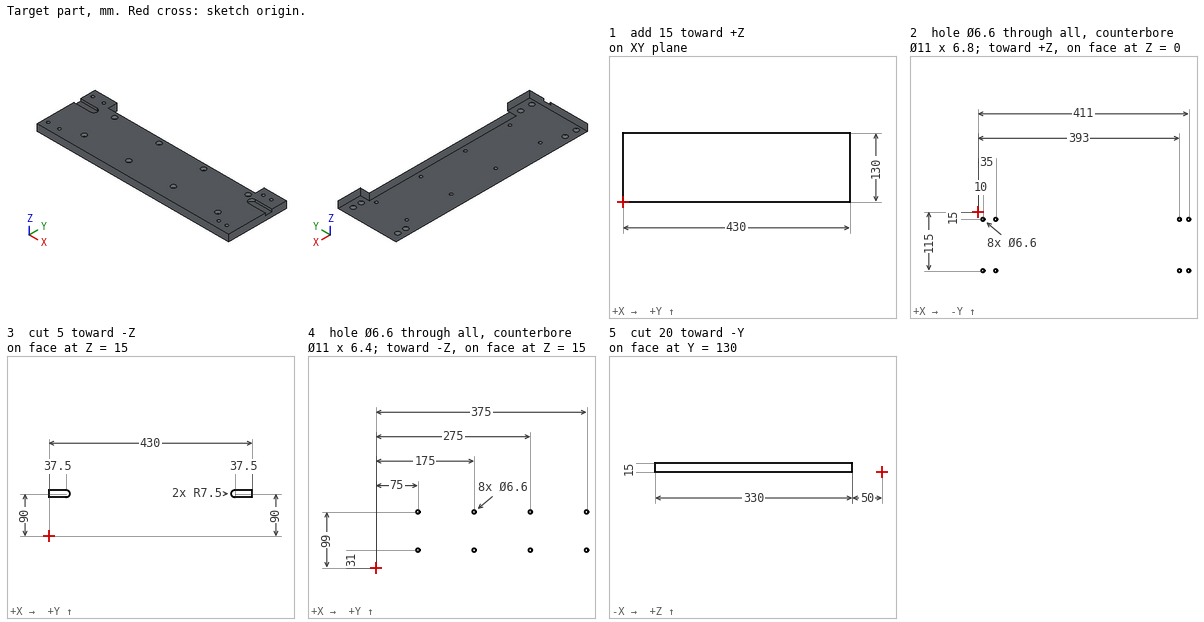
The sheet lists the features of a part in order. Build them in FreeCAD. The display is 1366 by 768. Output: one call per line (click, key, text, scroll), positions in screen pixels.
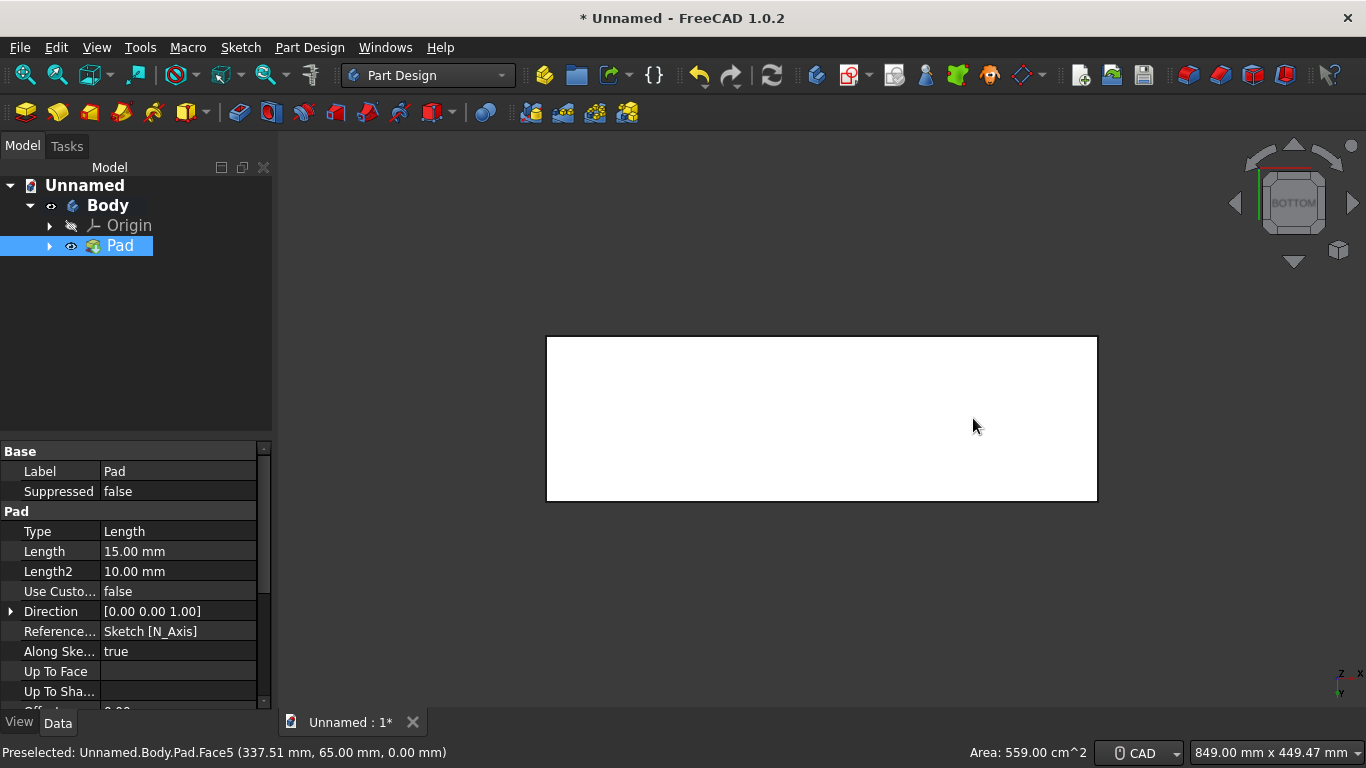
click(850, 76)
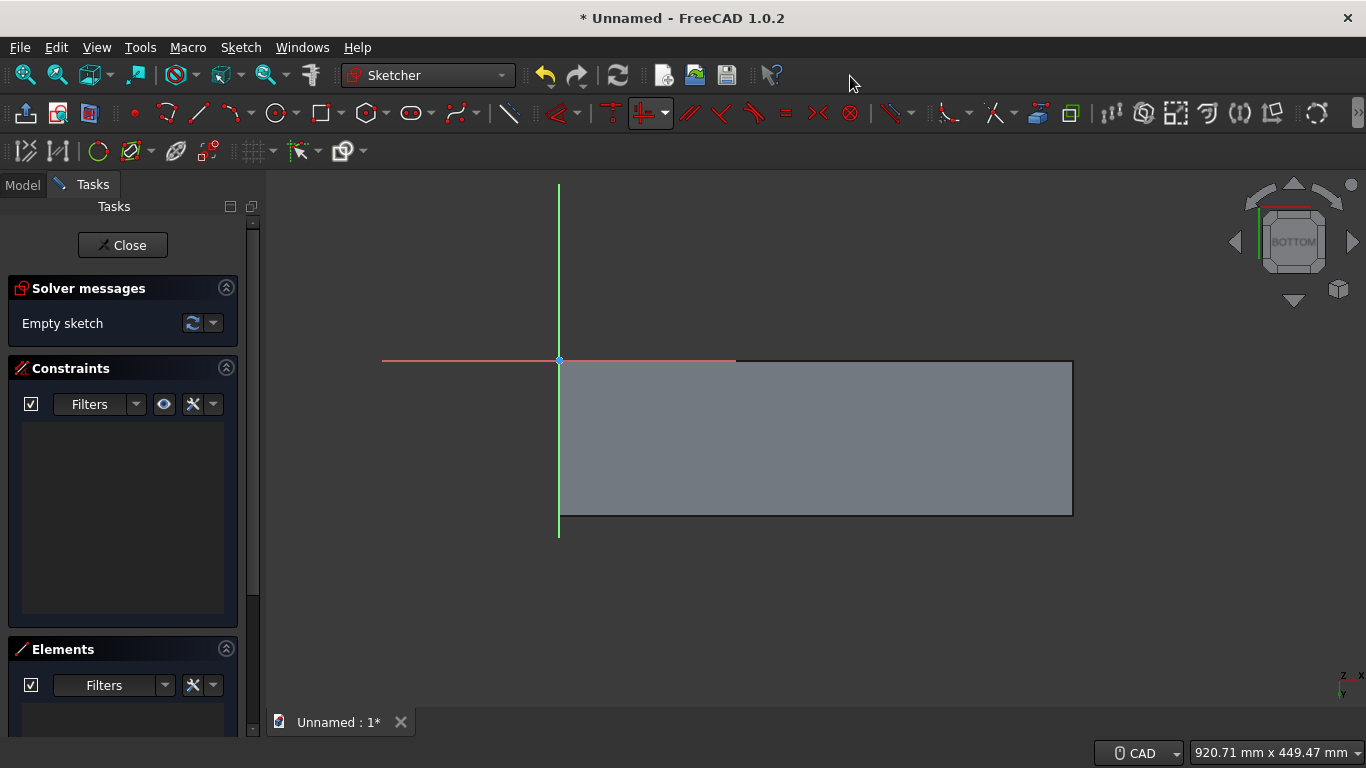
click(276, 114)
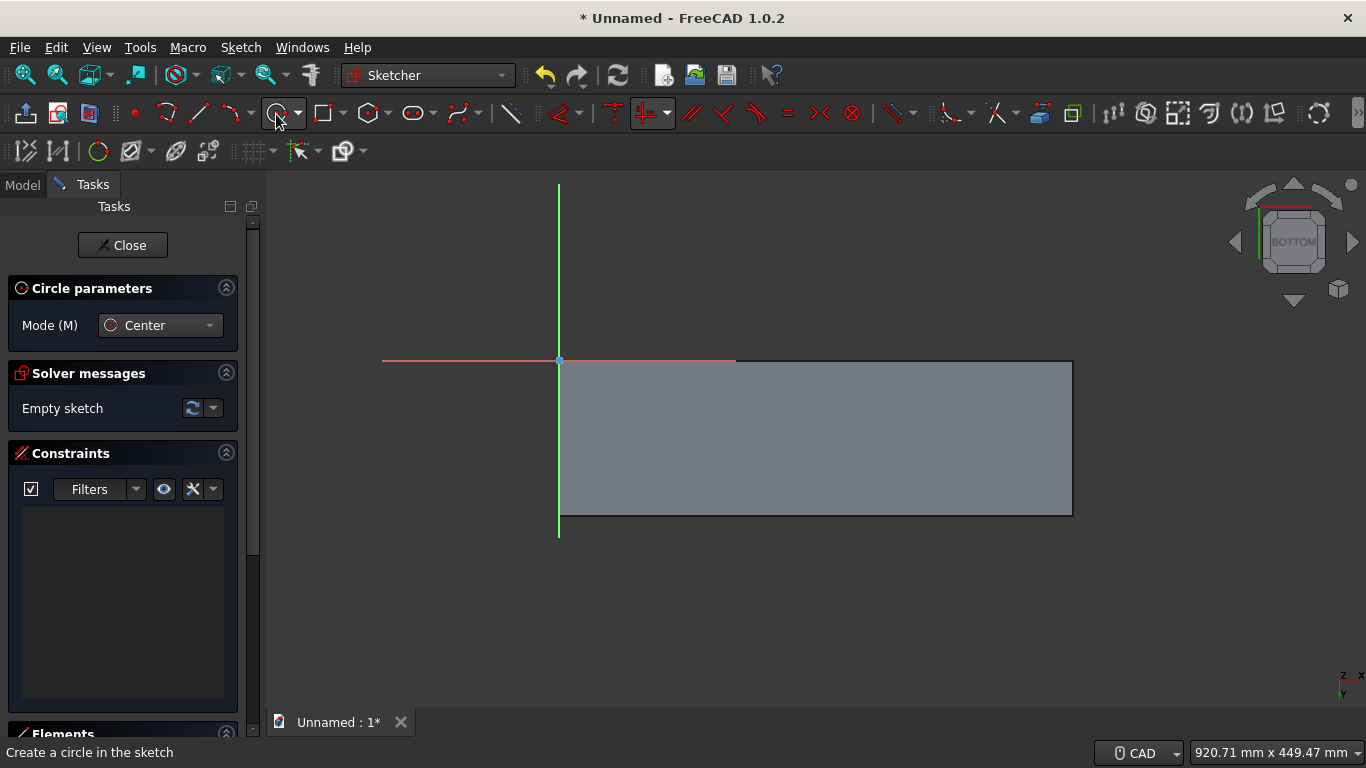
scroll(571, 379, up, 9)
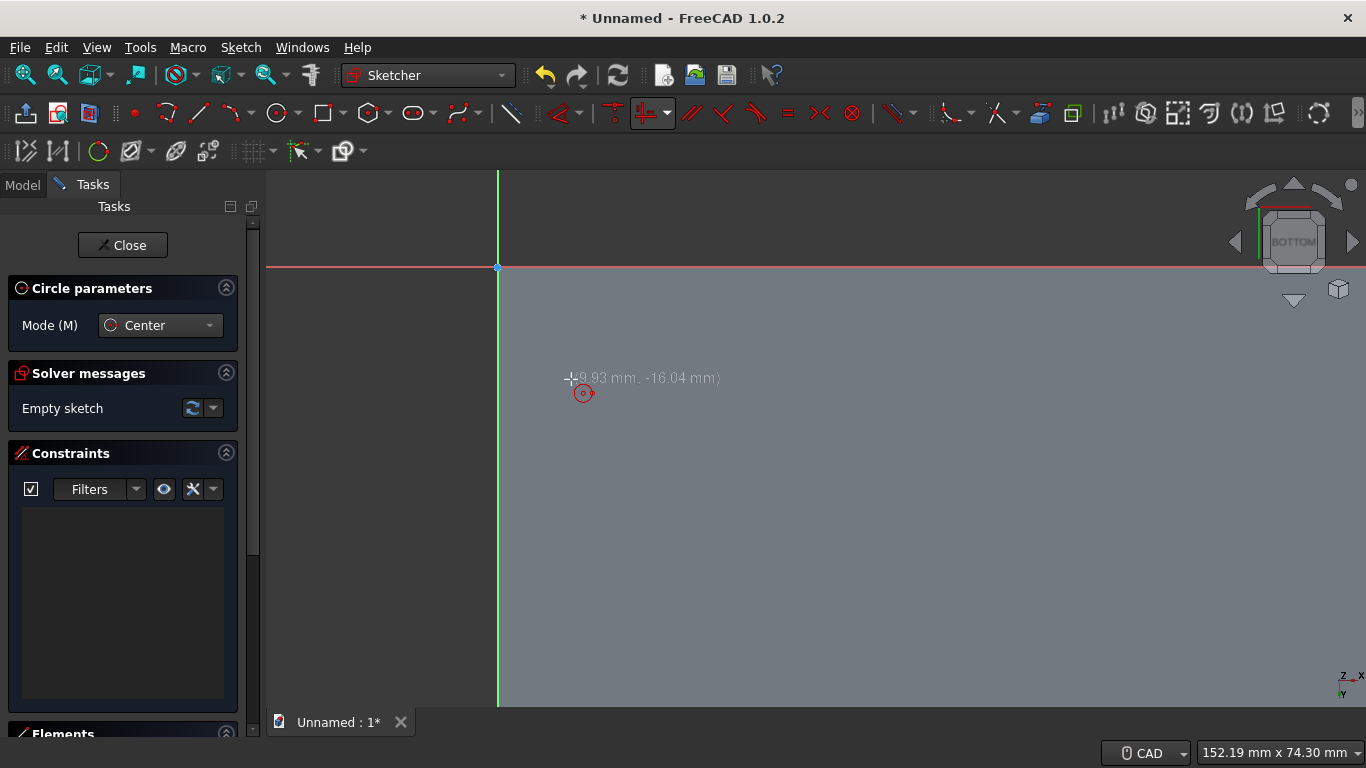
scroll(432, 374, down, 8)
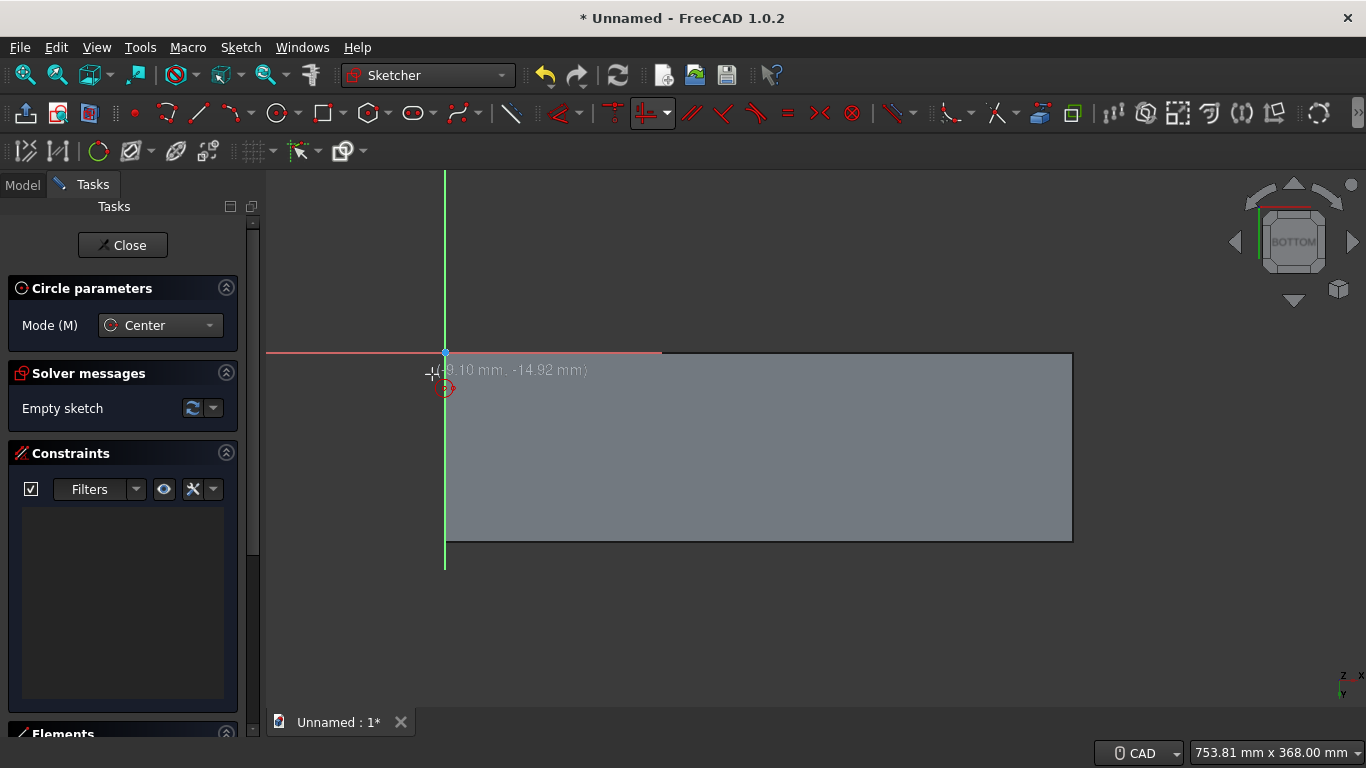
click(460, 375)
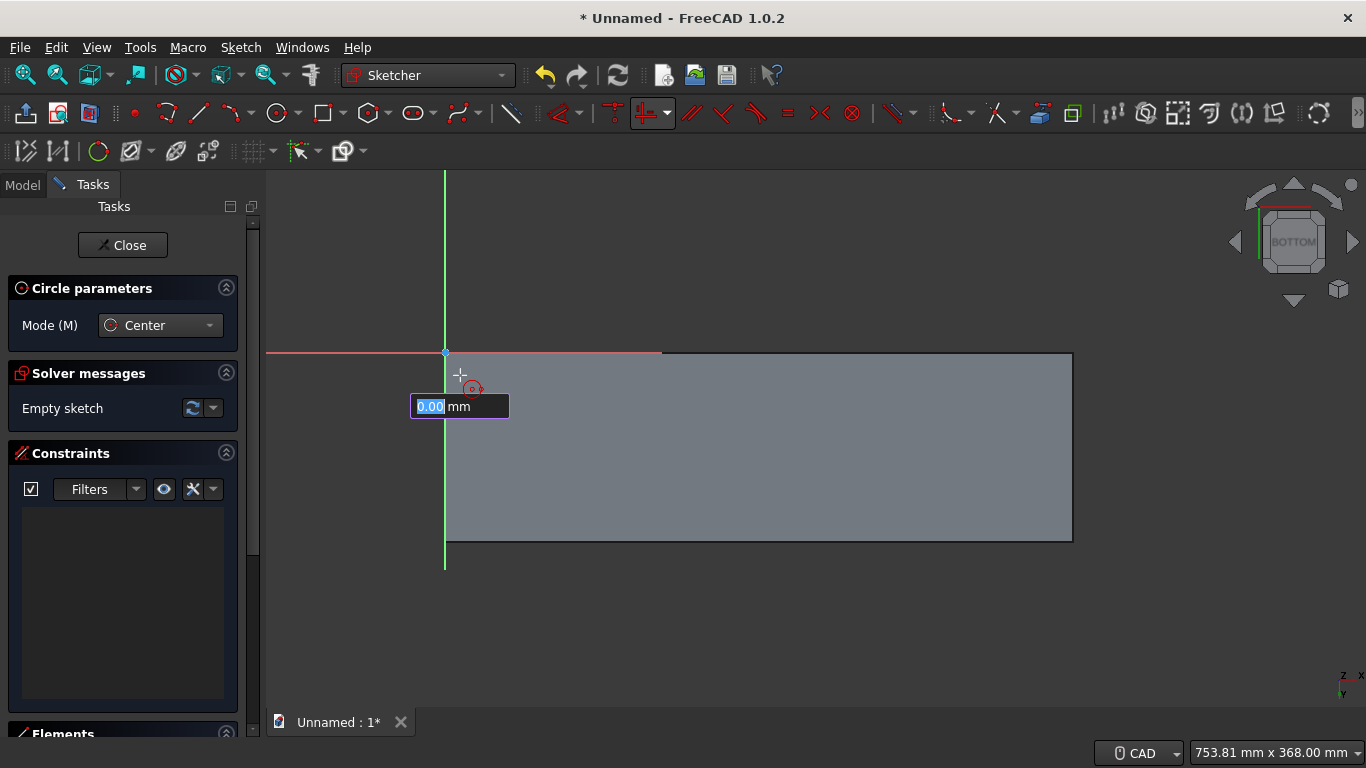
scroll(463, 371, up, 6)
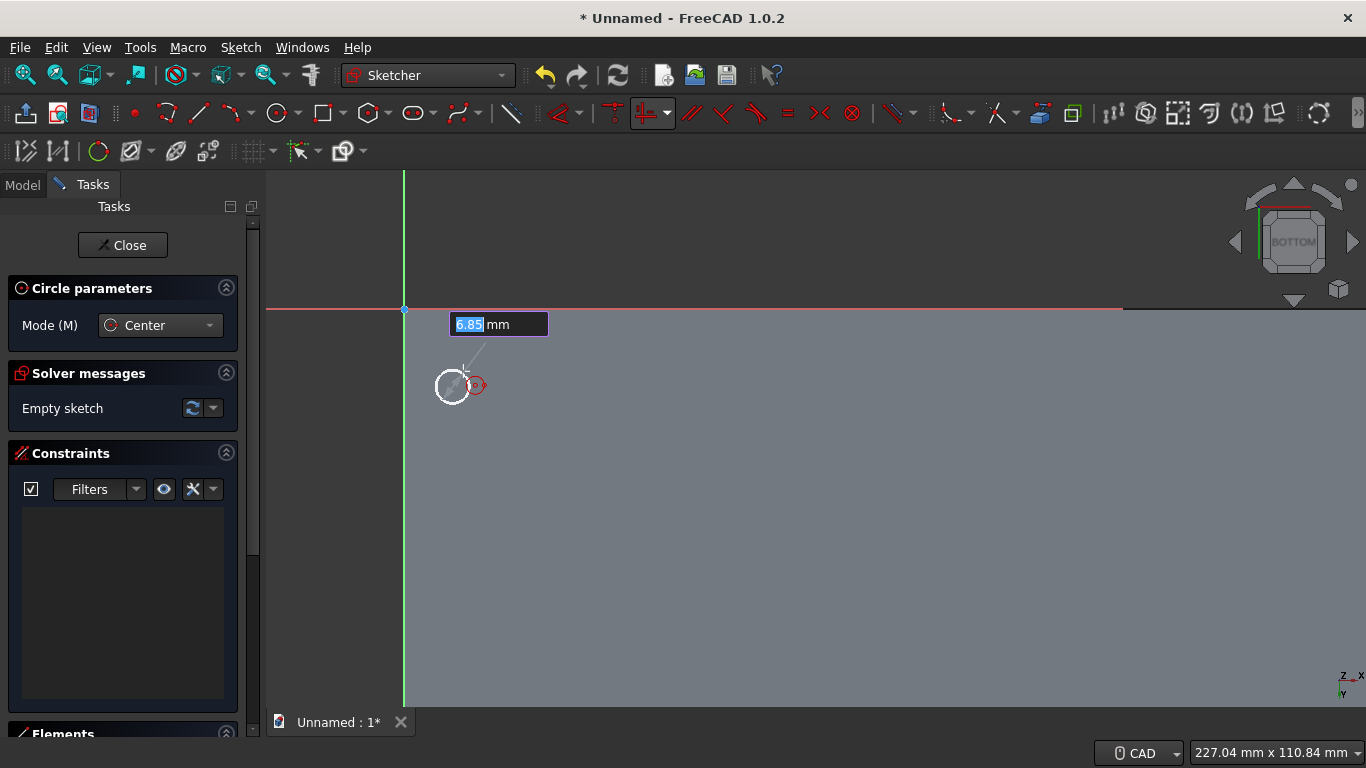
click(464, 371)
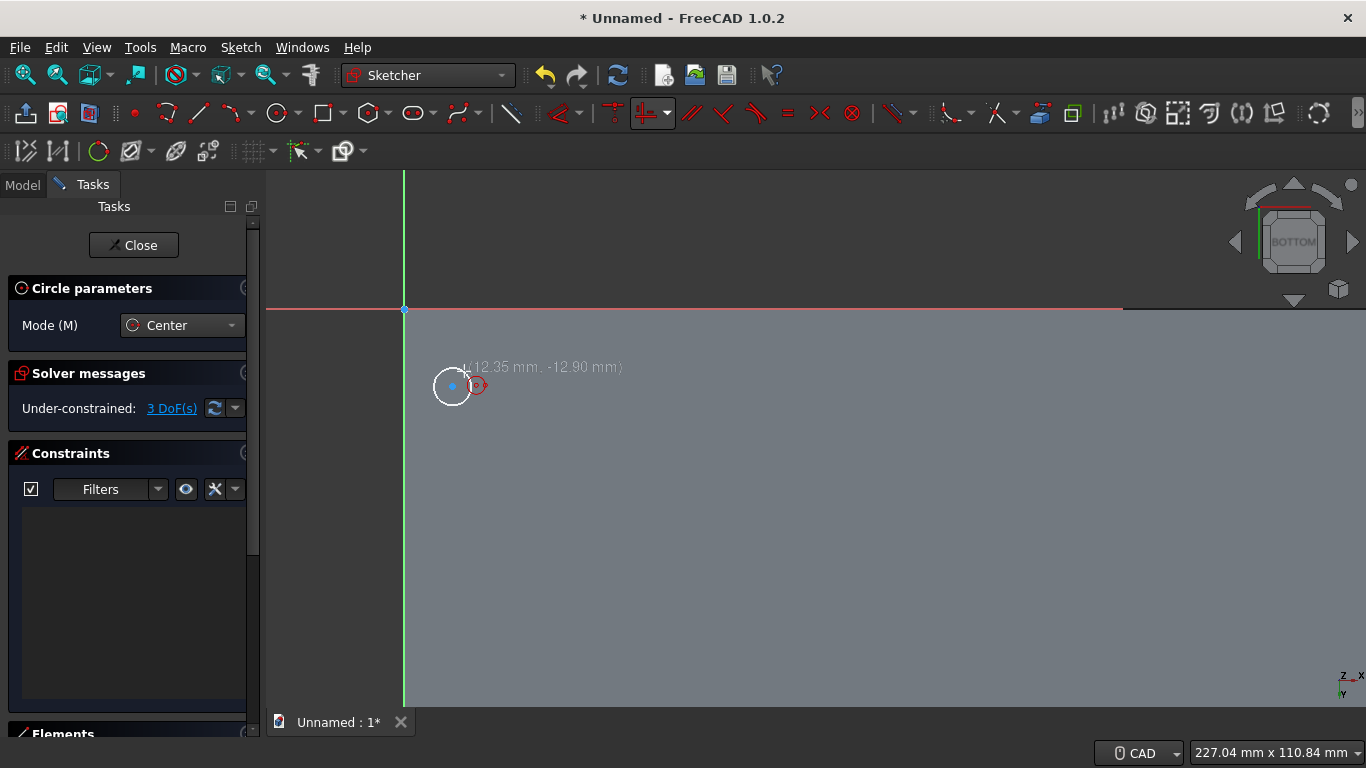
scroll(463, 371, down, 6)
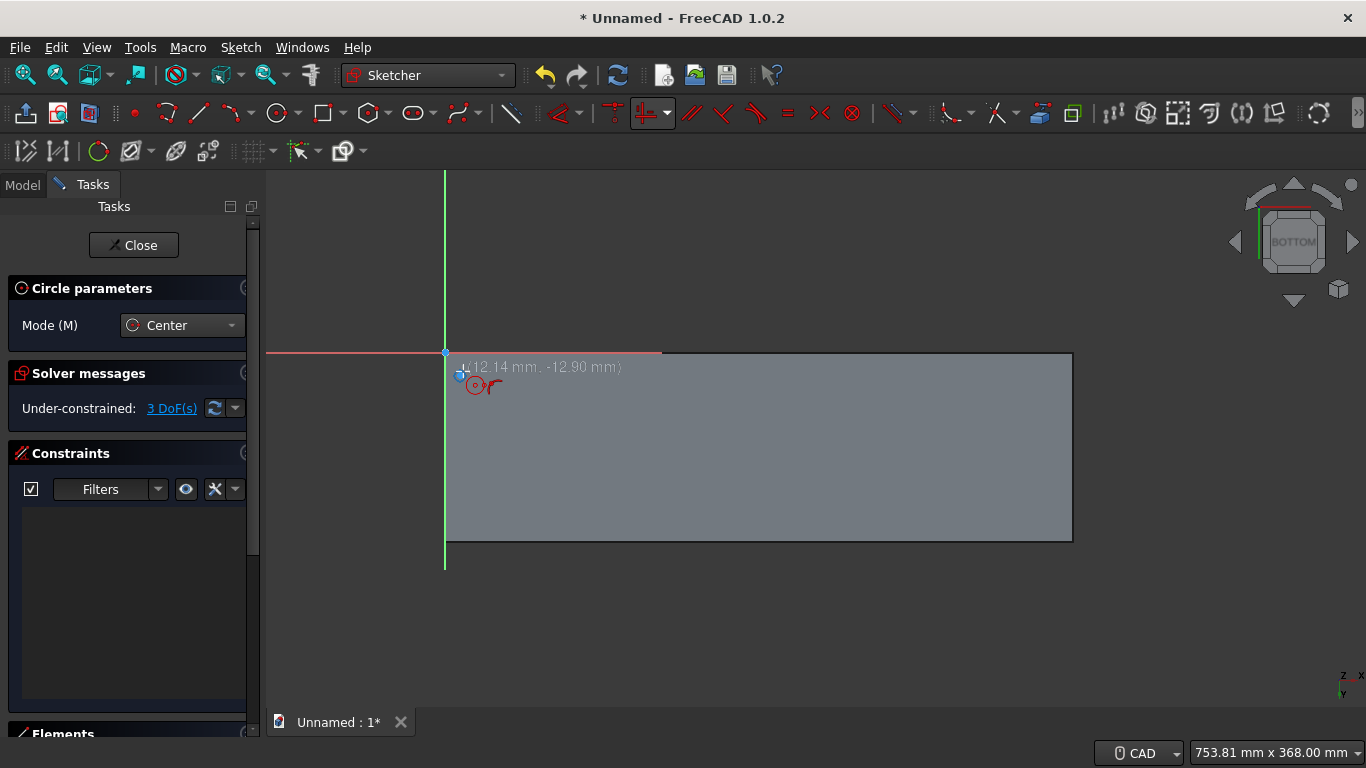
scroll(460, 521, up, 8)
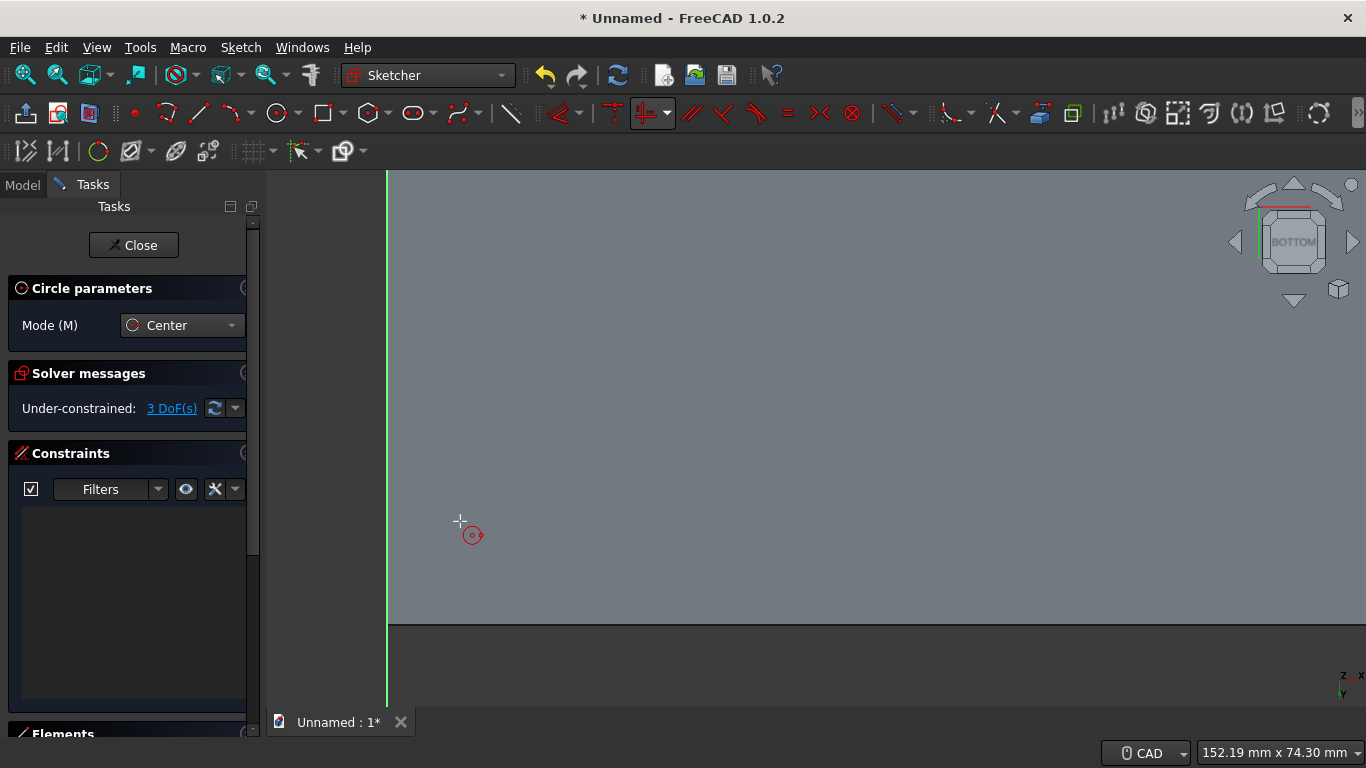
scroll(460, 521, down, 8)